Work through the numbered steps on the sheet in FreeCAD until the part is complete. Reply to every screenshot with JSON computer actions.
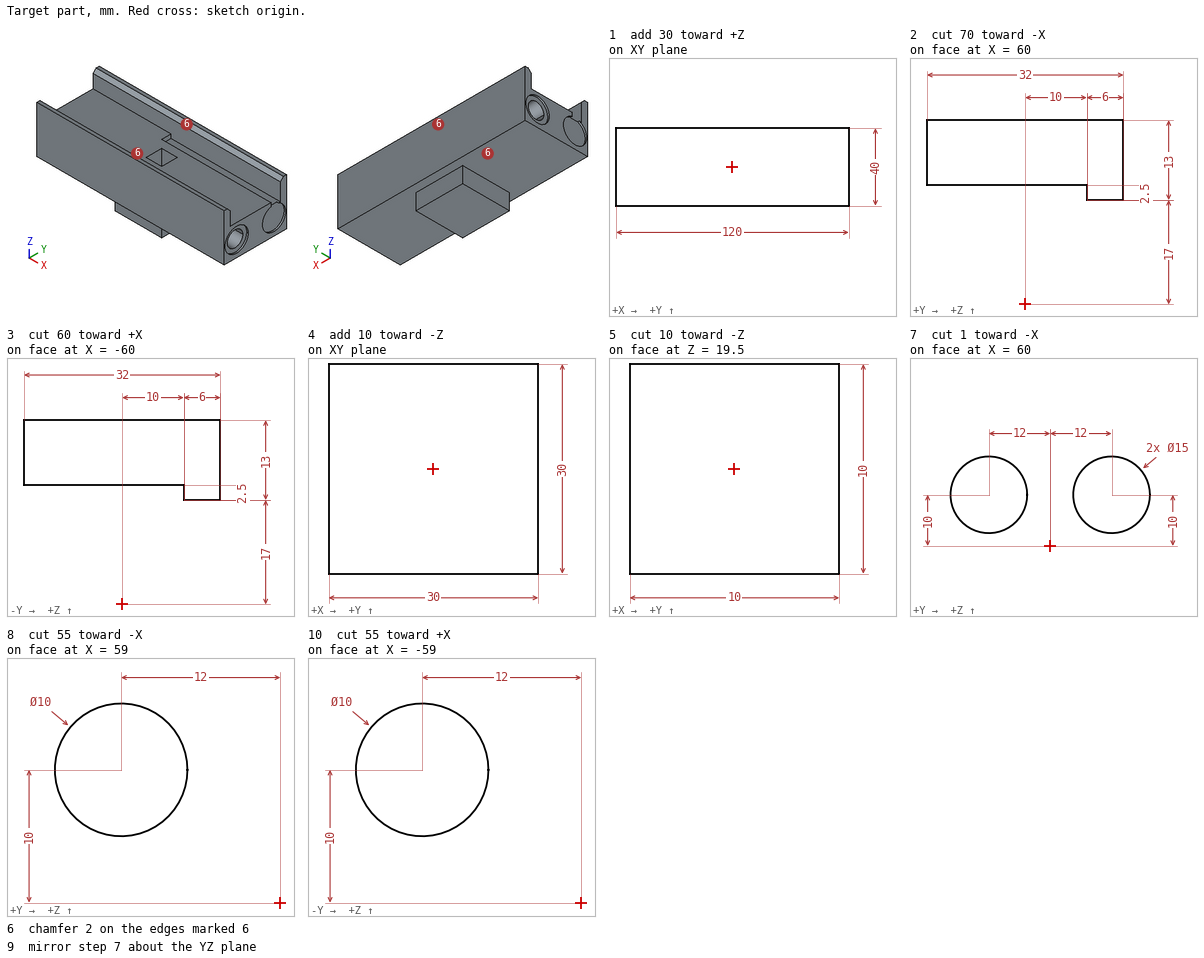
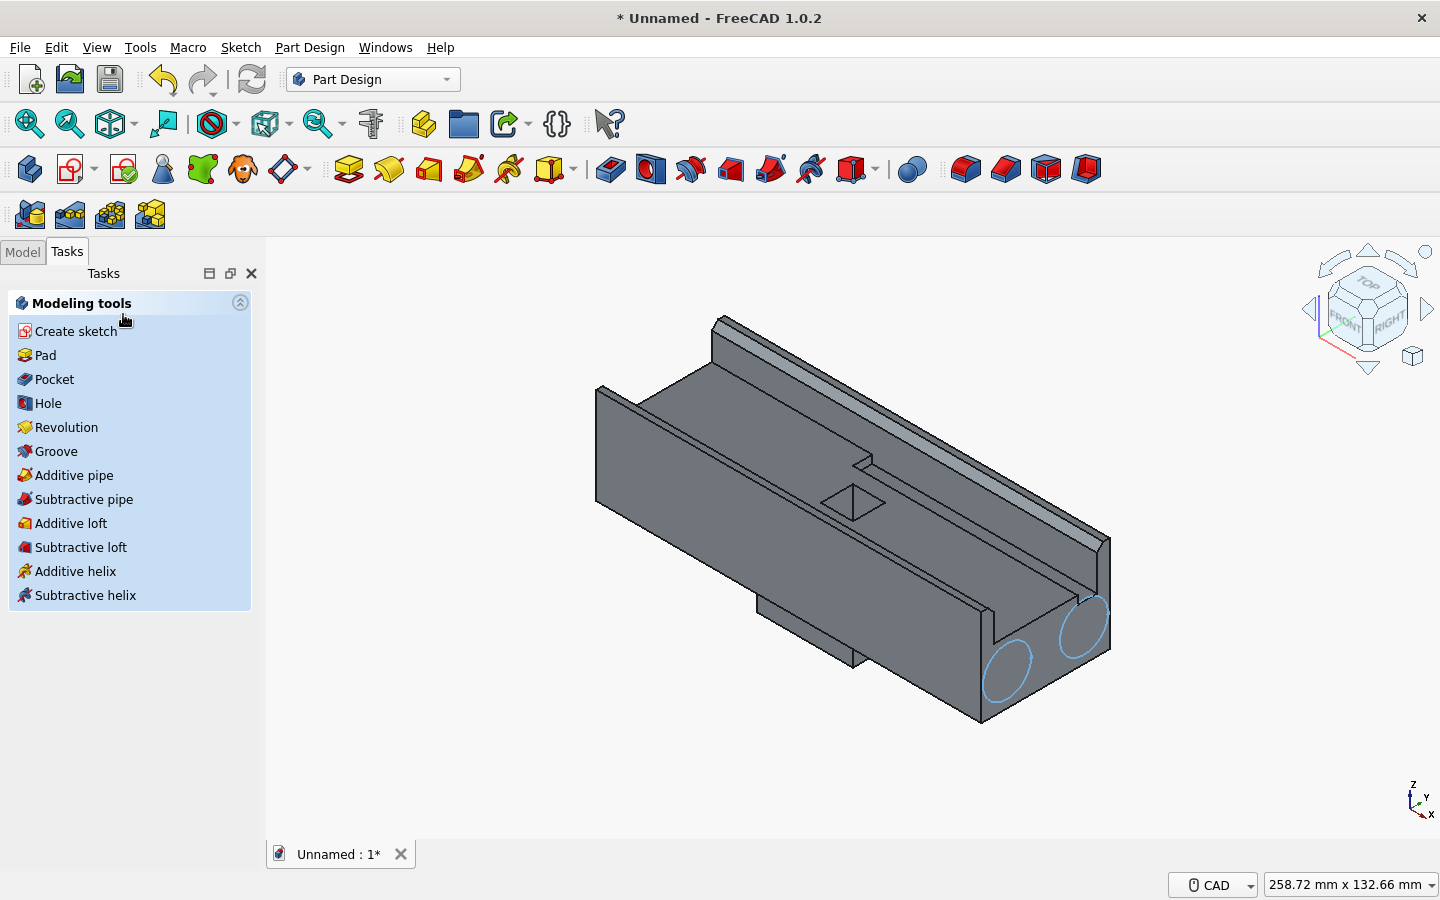
{"action": "left_click", "coordinate": [612, 170]}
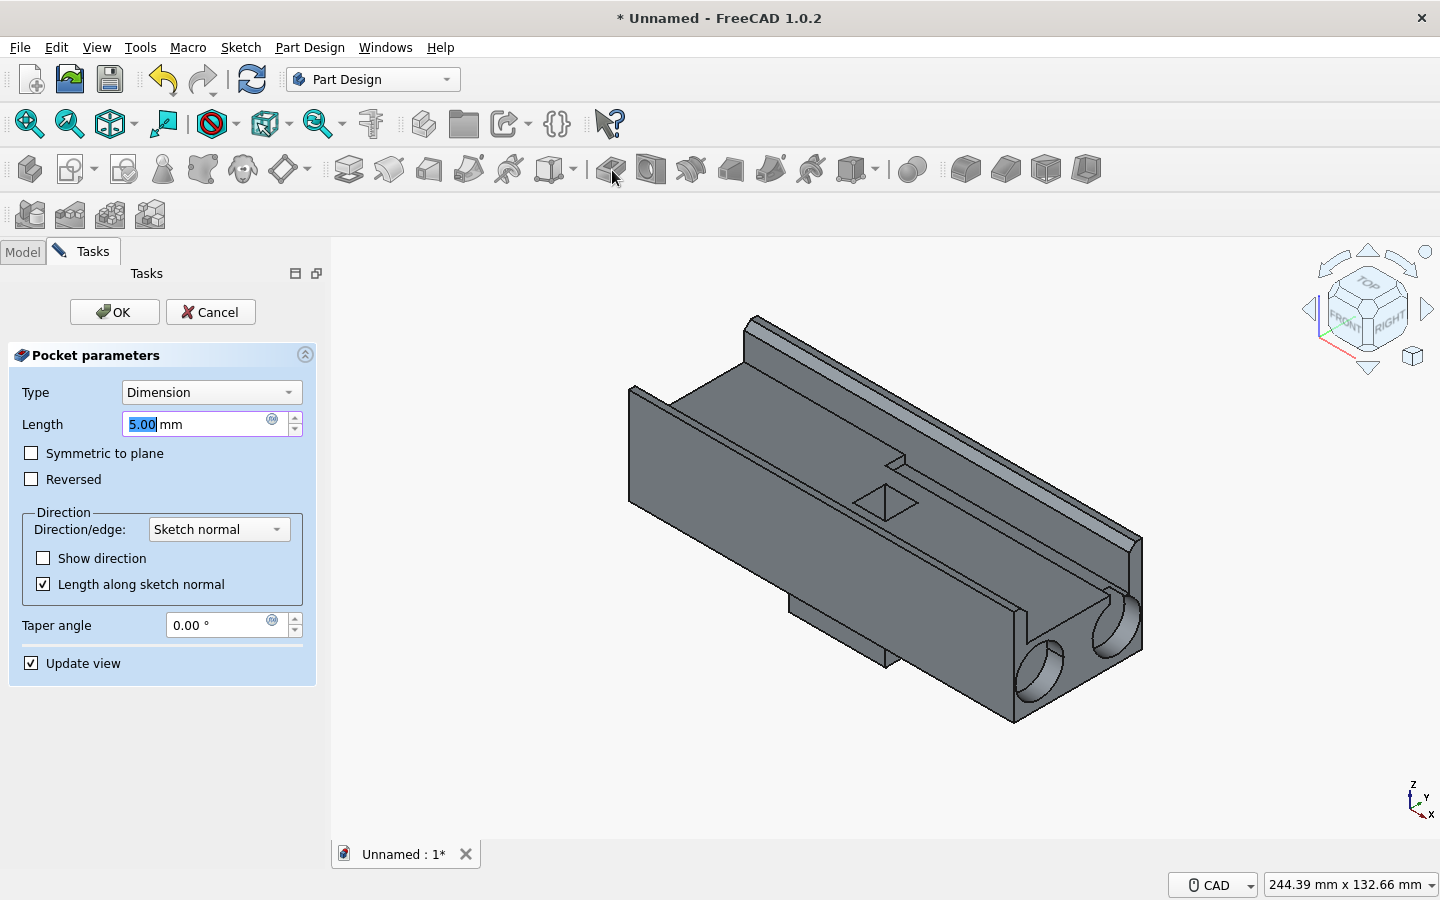
{"action": "type", "text": "1"}
{"action": "key", "text": "Tab"}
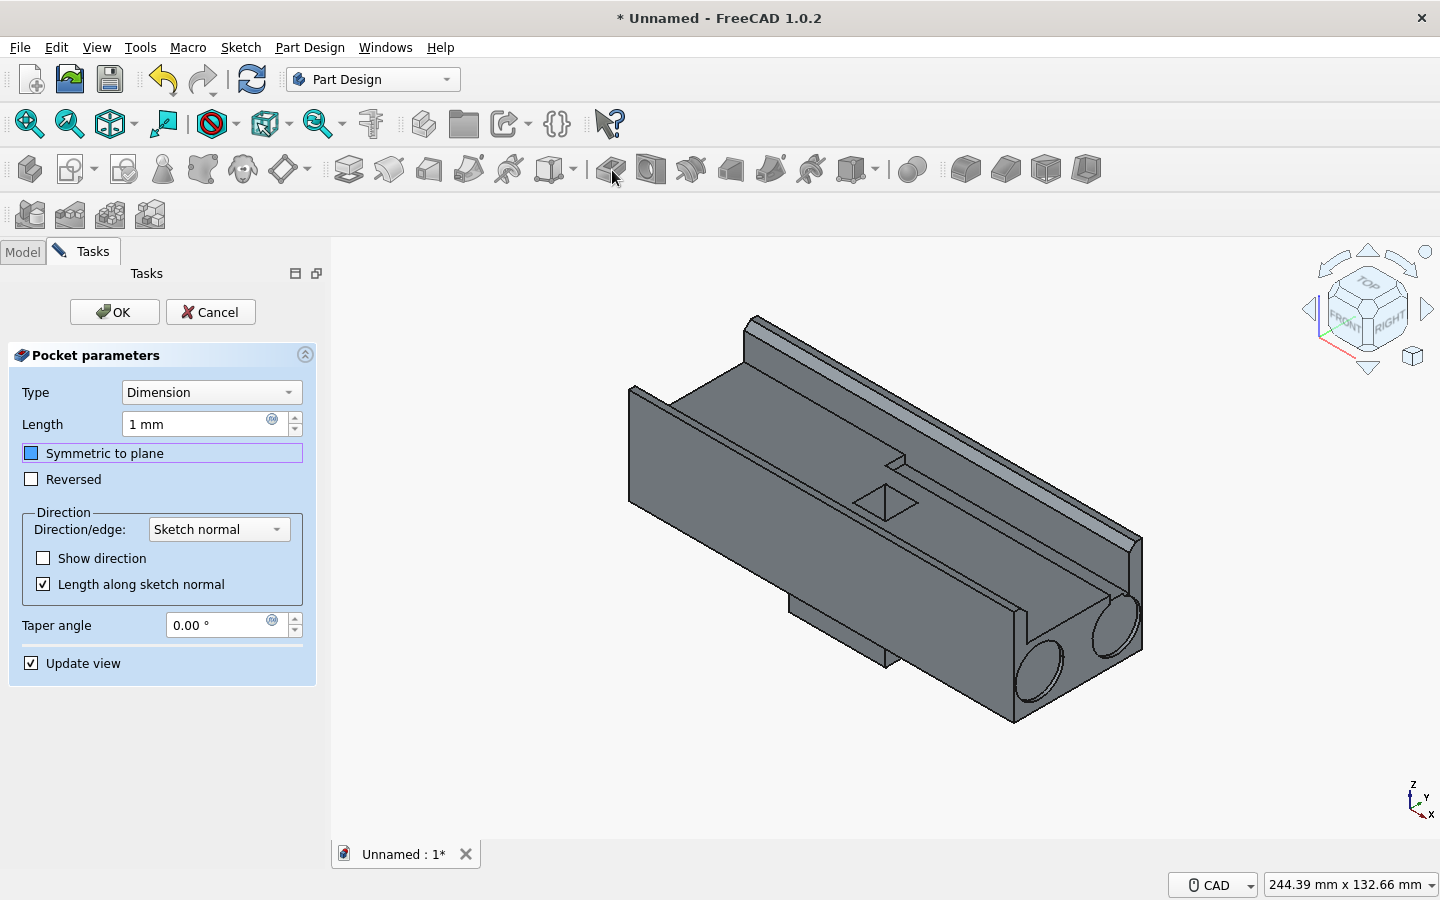
{"action": "left_click", "coordinate": [115, 312]}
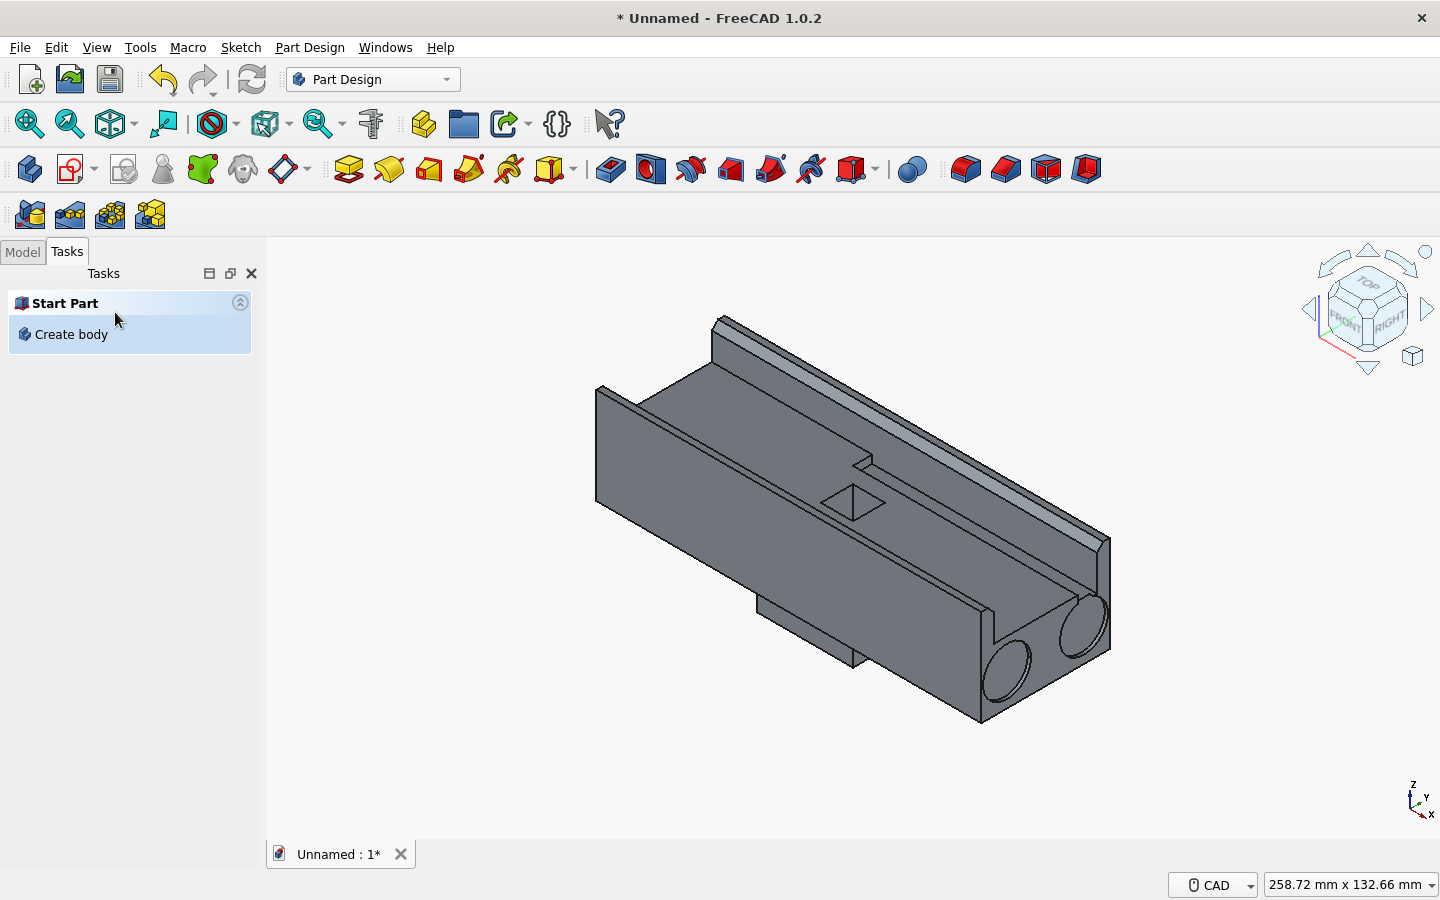
{"action": "left_click", "coordinate": [1004, 669]}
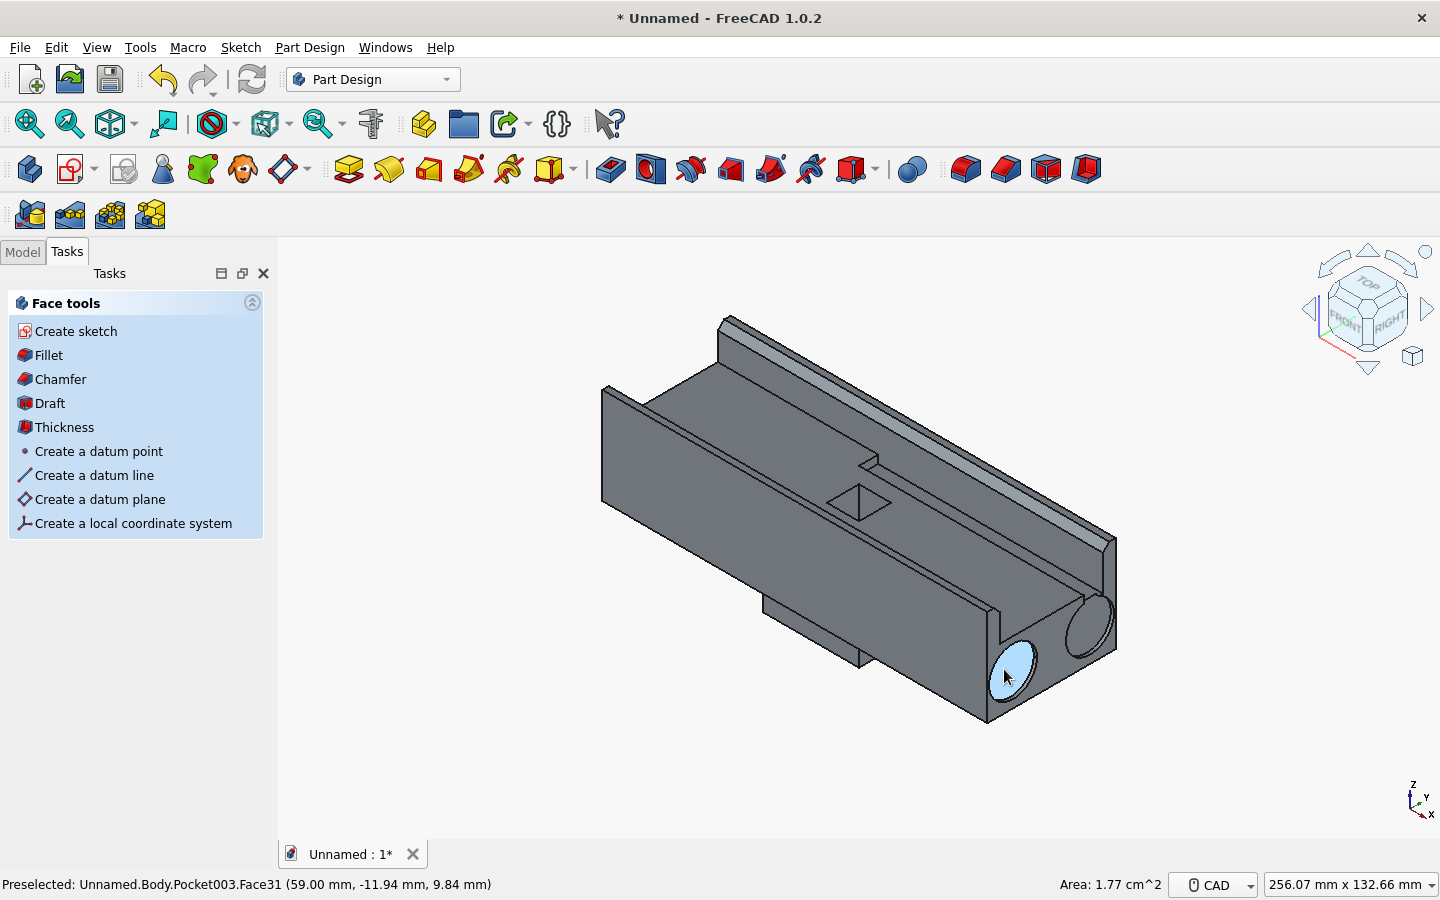
{"action": "left_click", "coordinate": [70, 170]}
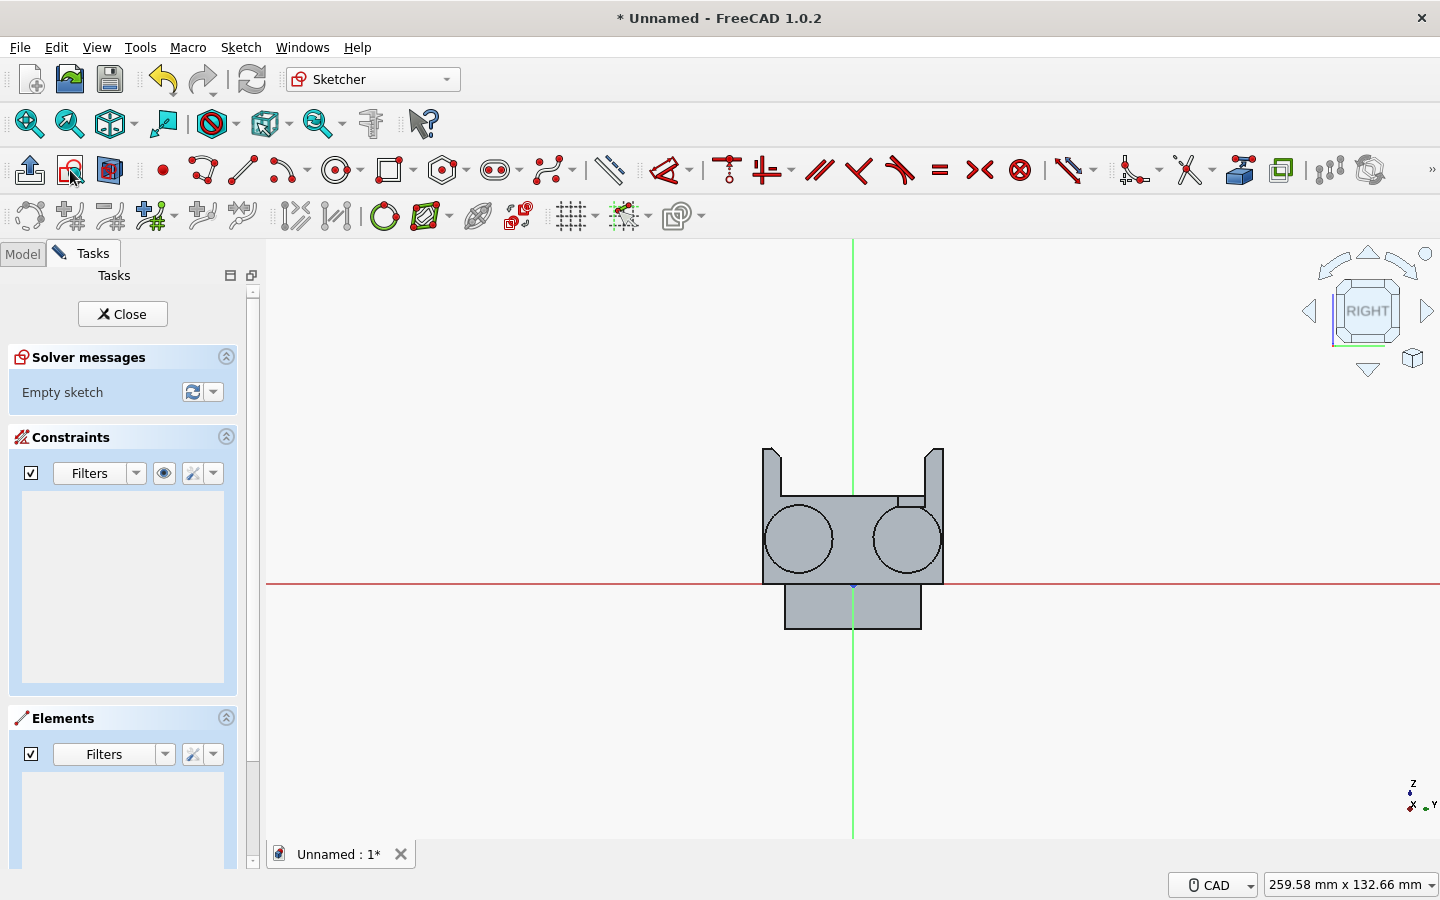
{"action": "scroll", "coordinate": [821, 553], "scroll_direction": "up", "scroll_amount": 9}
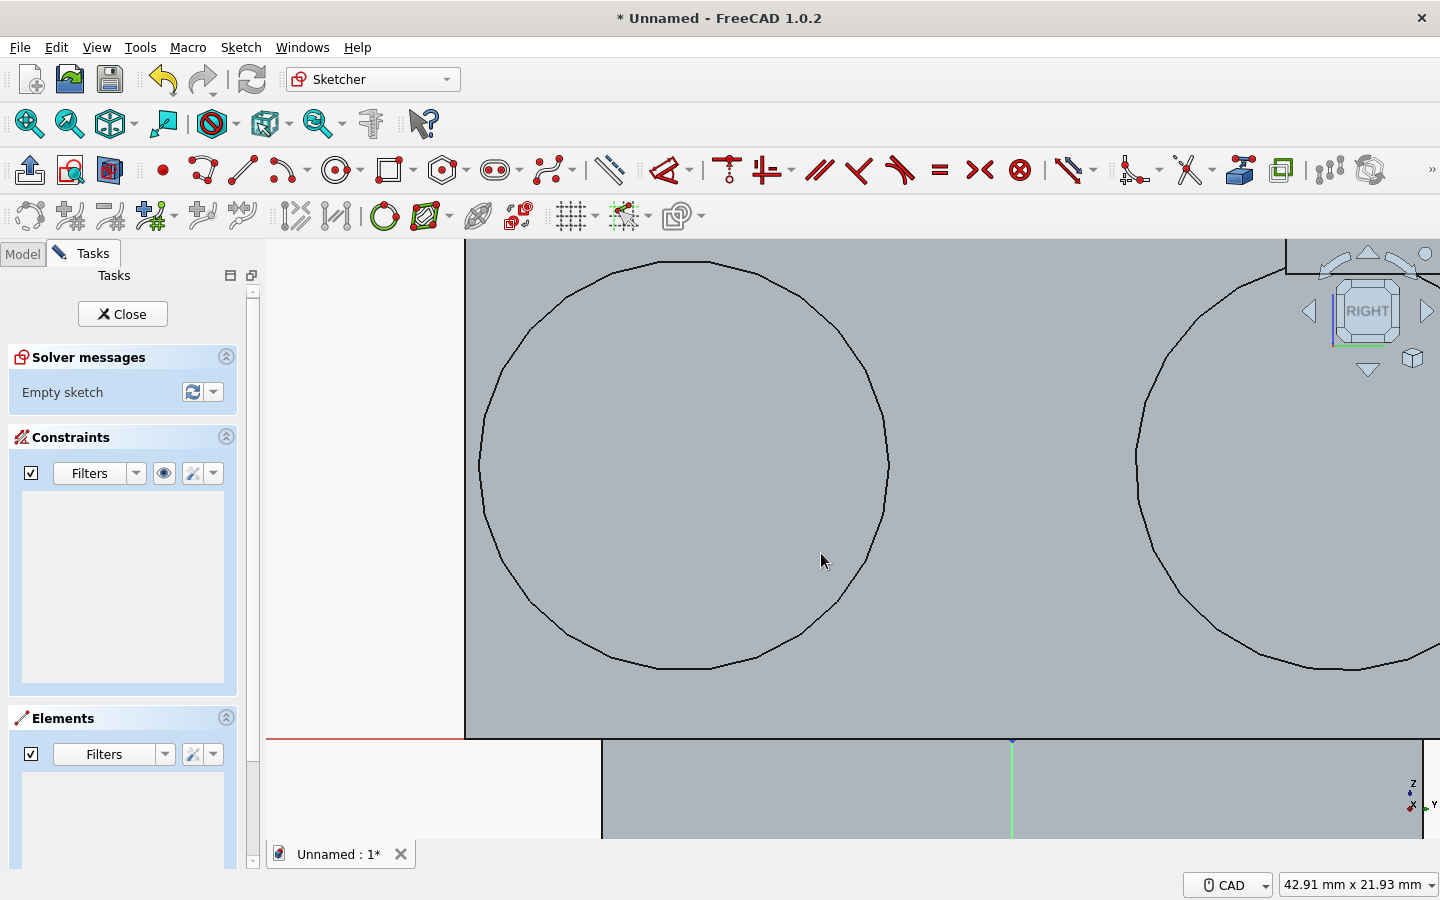
{"action": "left_click", "coordinate": [336, 170]}